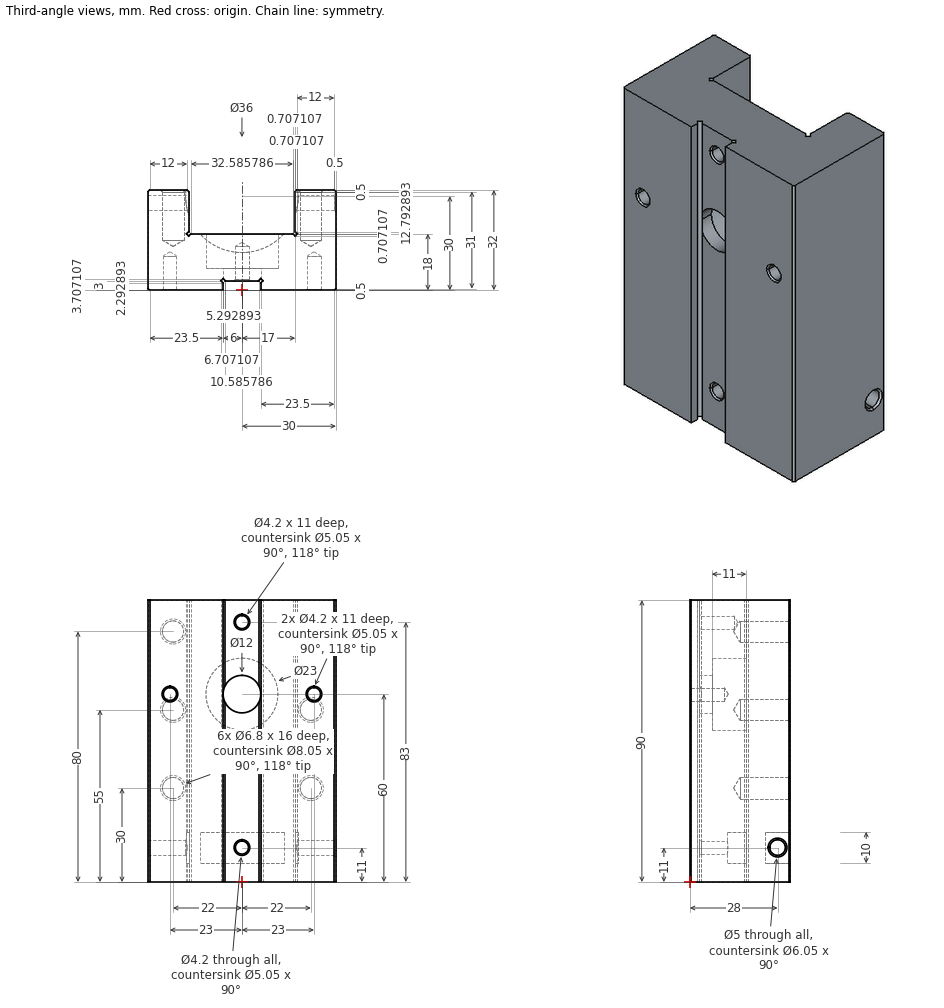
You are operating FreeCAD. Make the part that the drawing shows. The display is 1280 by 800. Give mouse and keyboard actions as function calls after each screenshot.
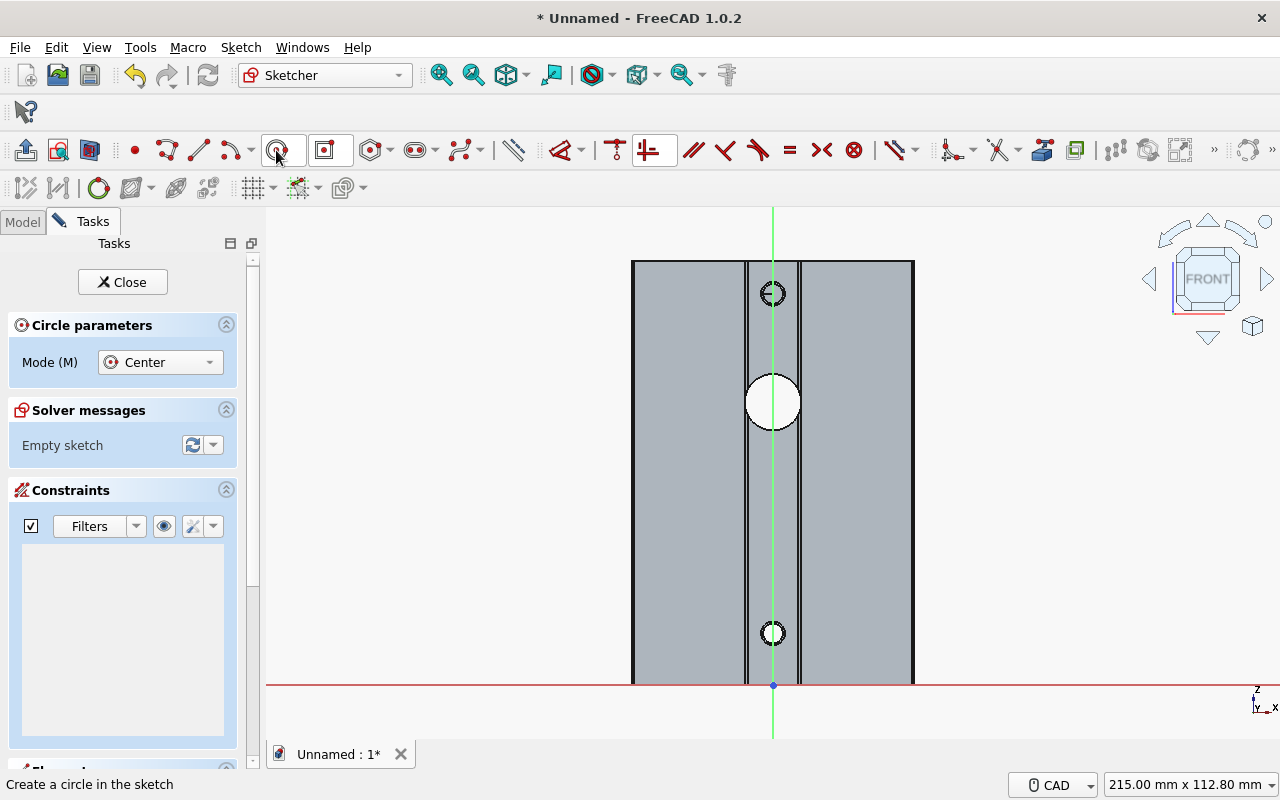
scroll(881, 402, up, 5)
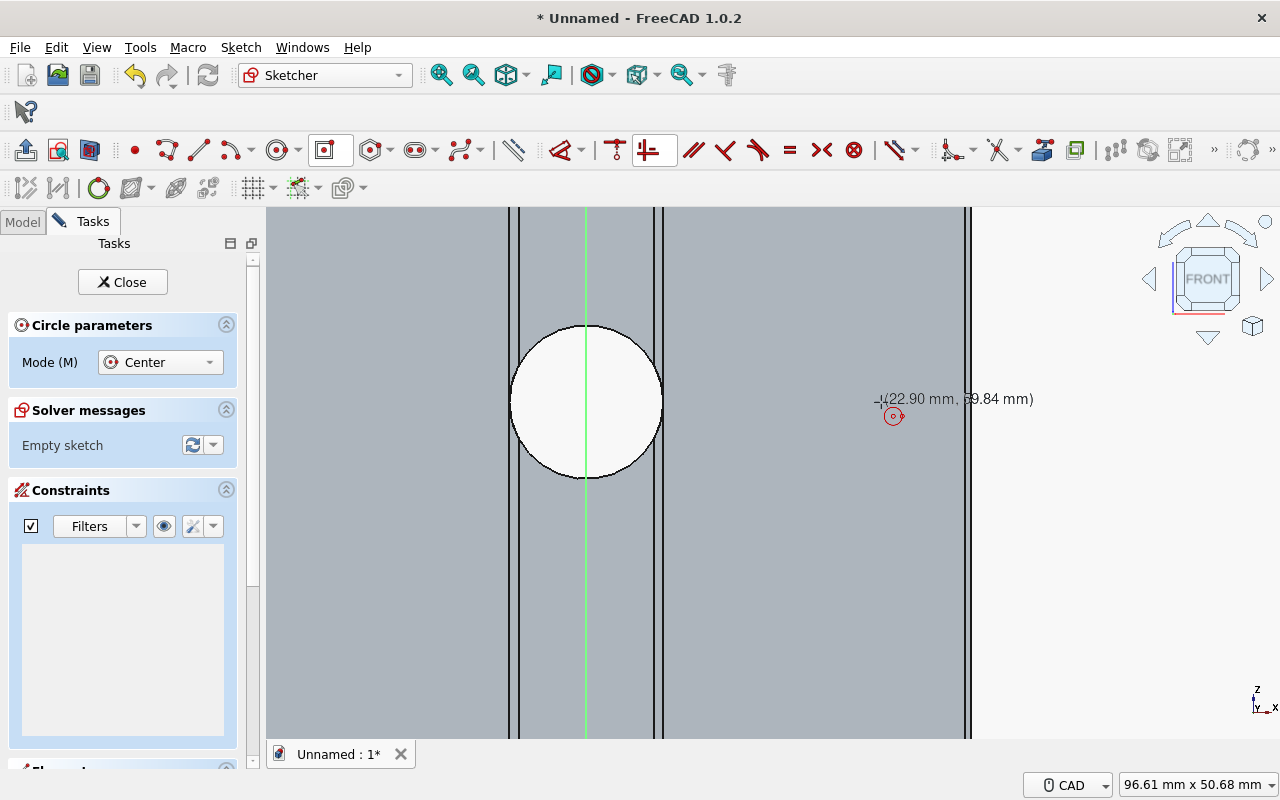
click(881, 402)
move(900, 383)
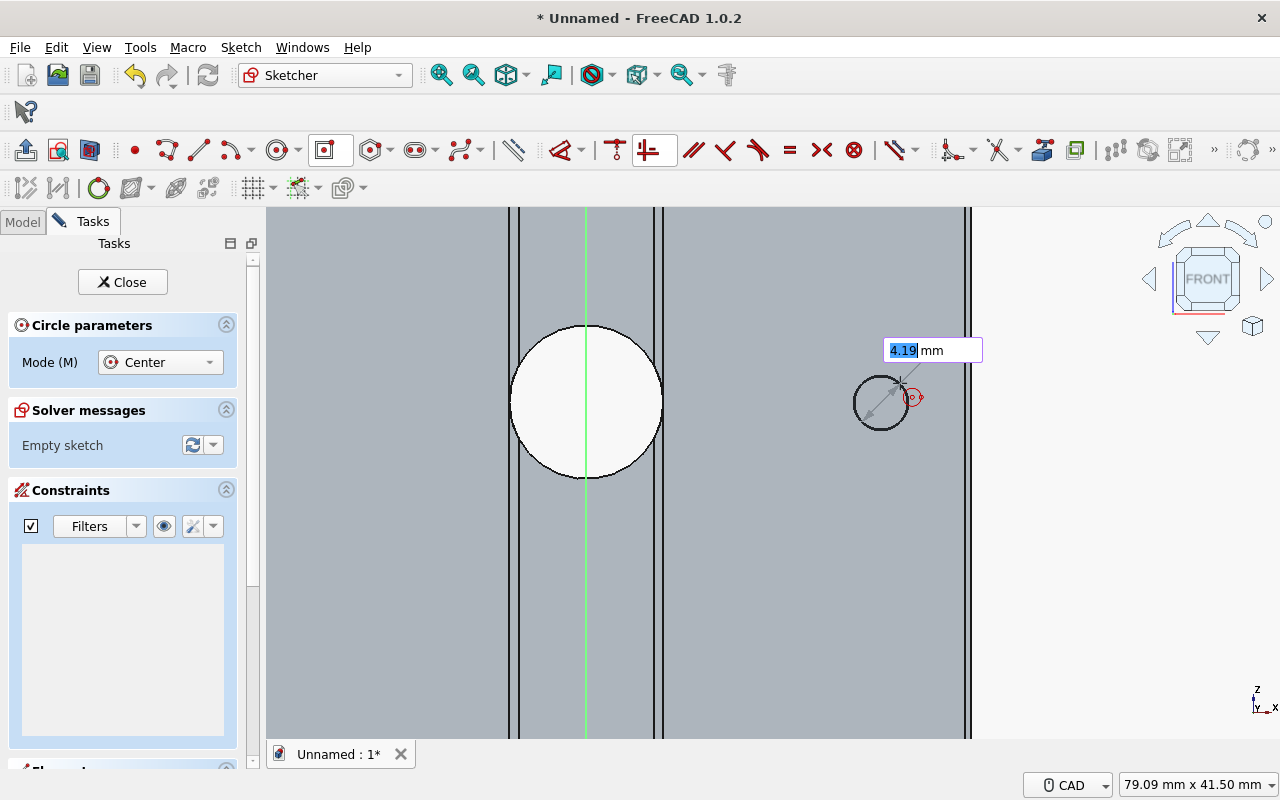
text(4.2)
key(Return)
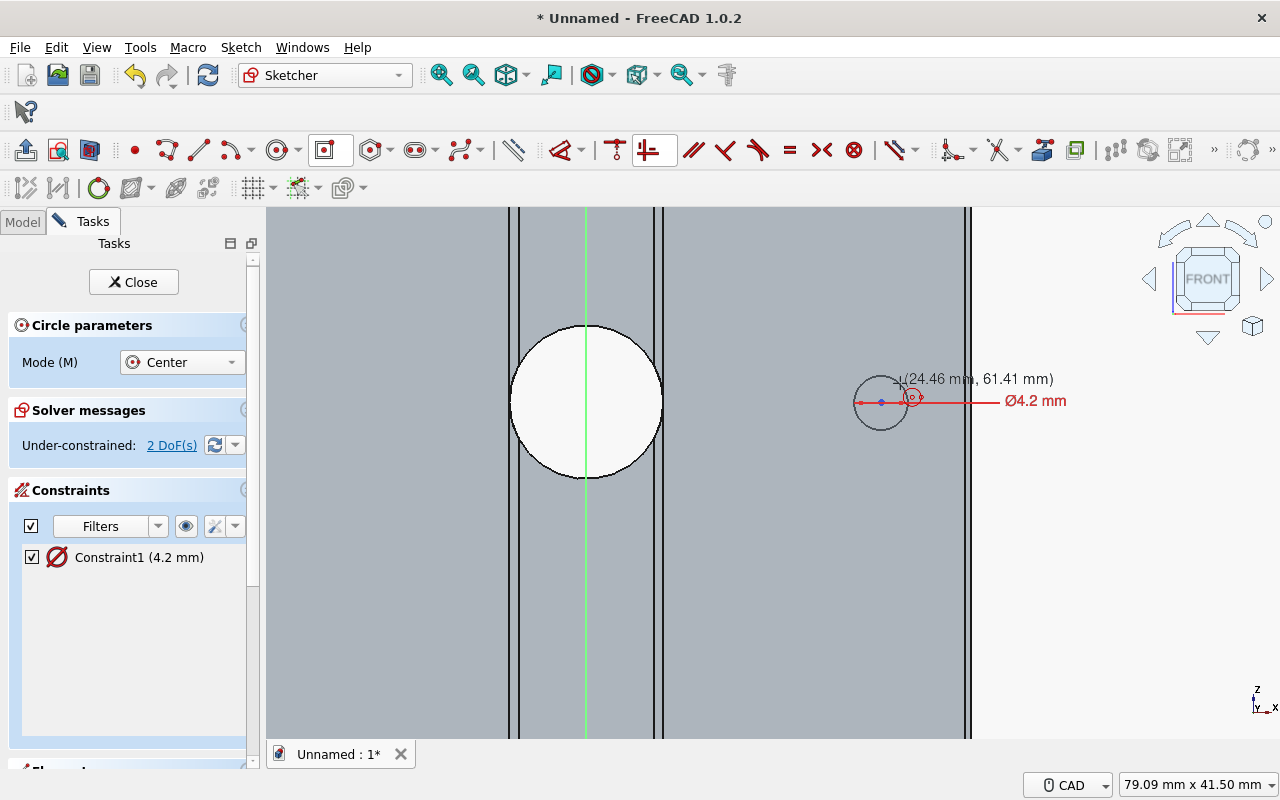
scroll(801, 235, down, 4)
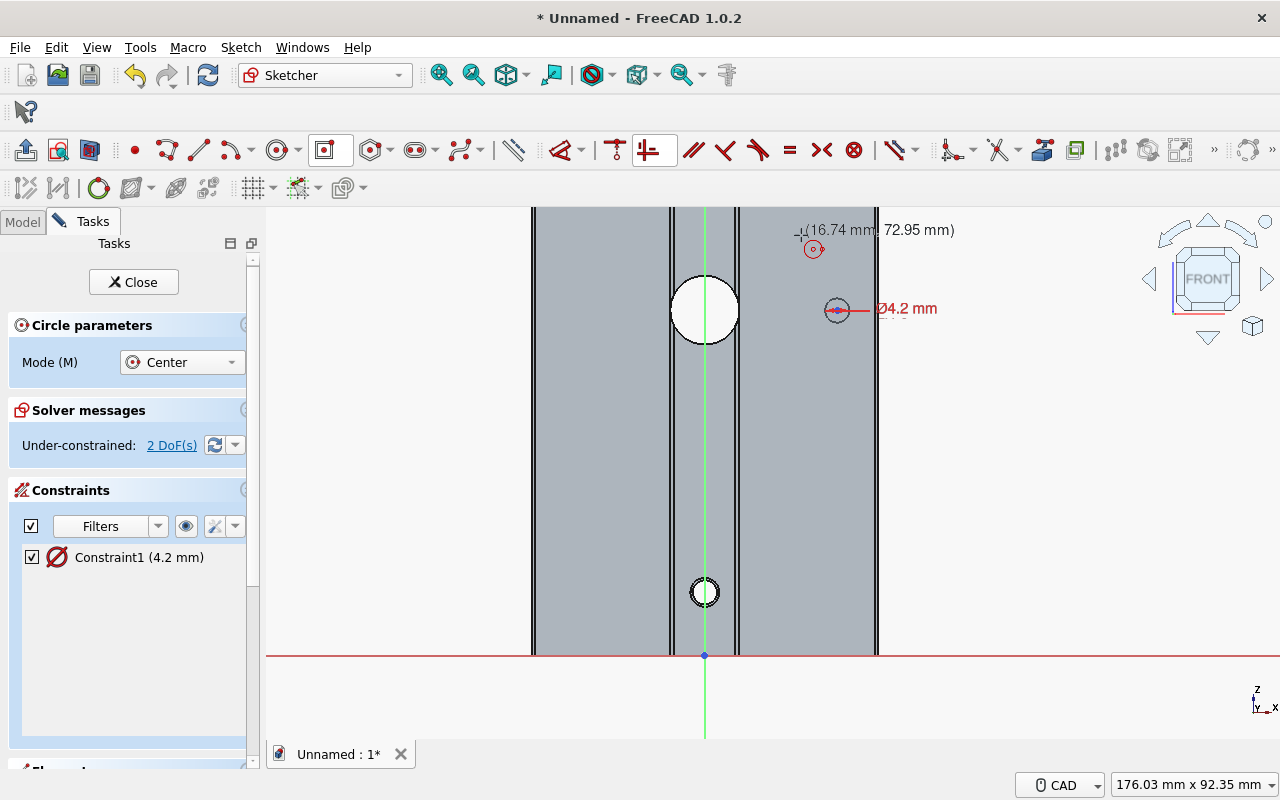
scroll(572, 310, up, 4)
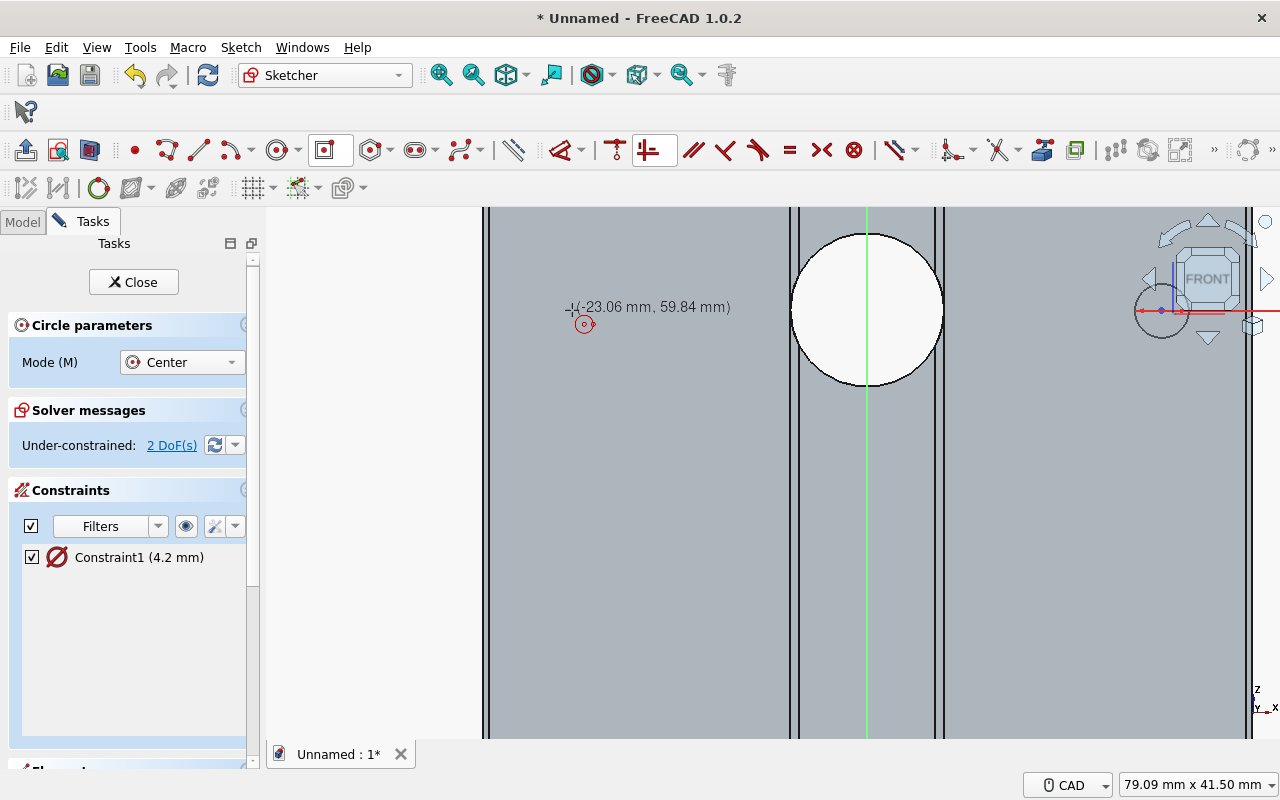
click(572, 310)
move(591, 291)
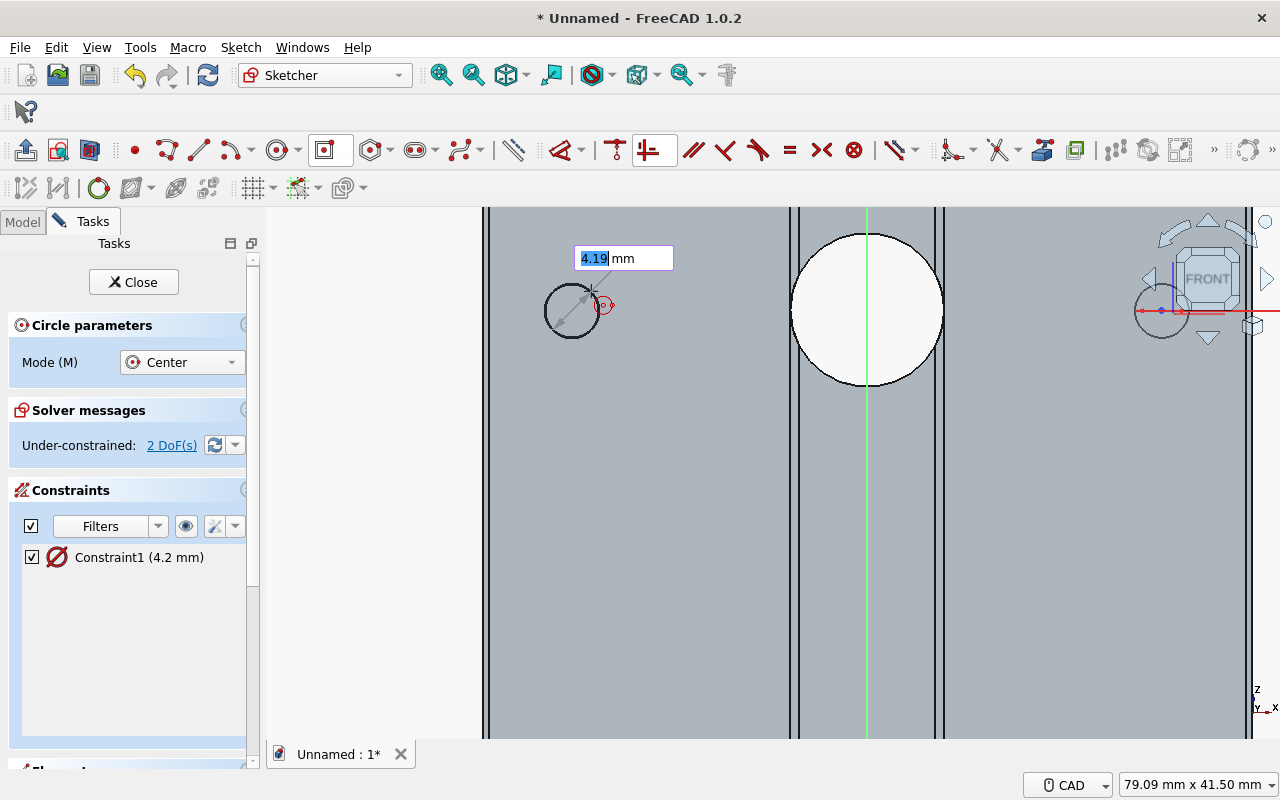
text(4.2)
key(Return)
key(Escape)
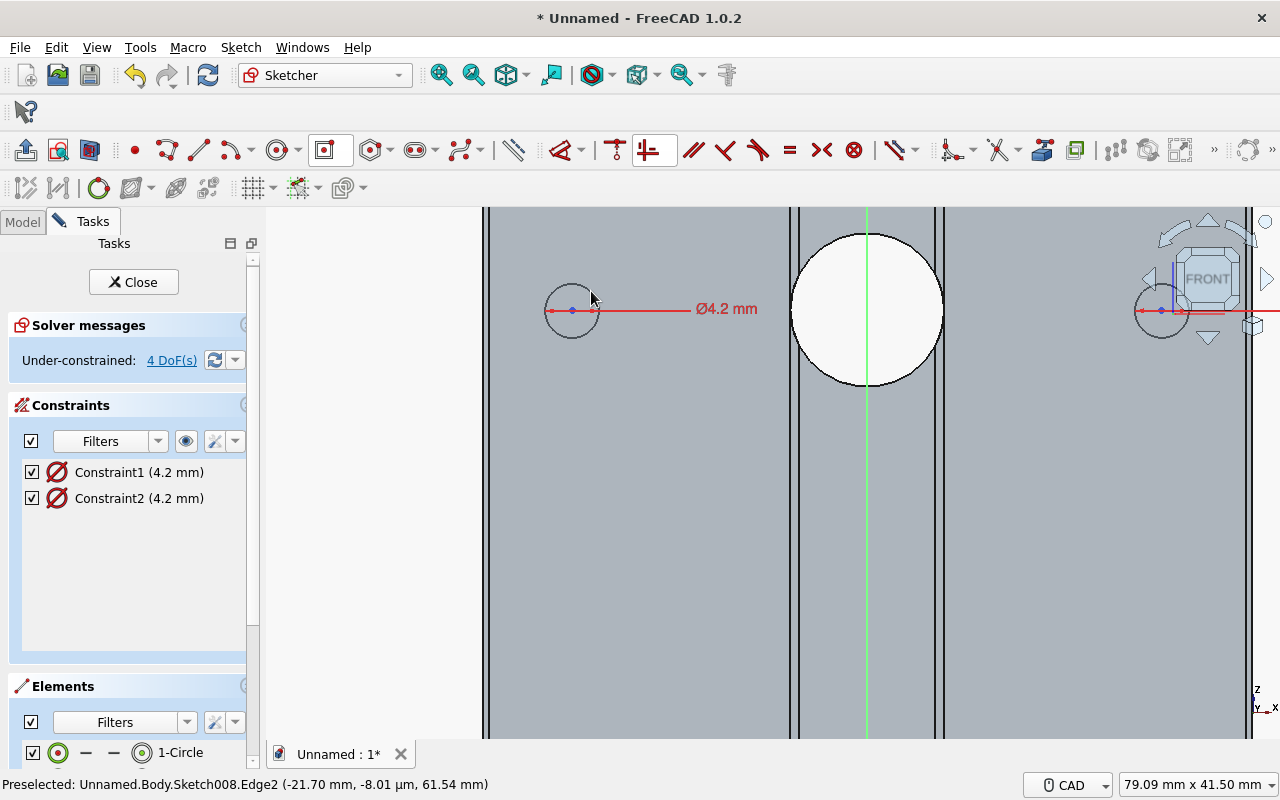
scroll(572, 303, down, 4)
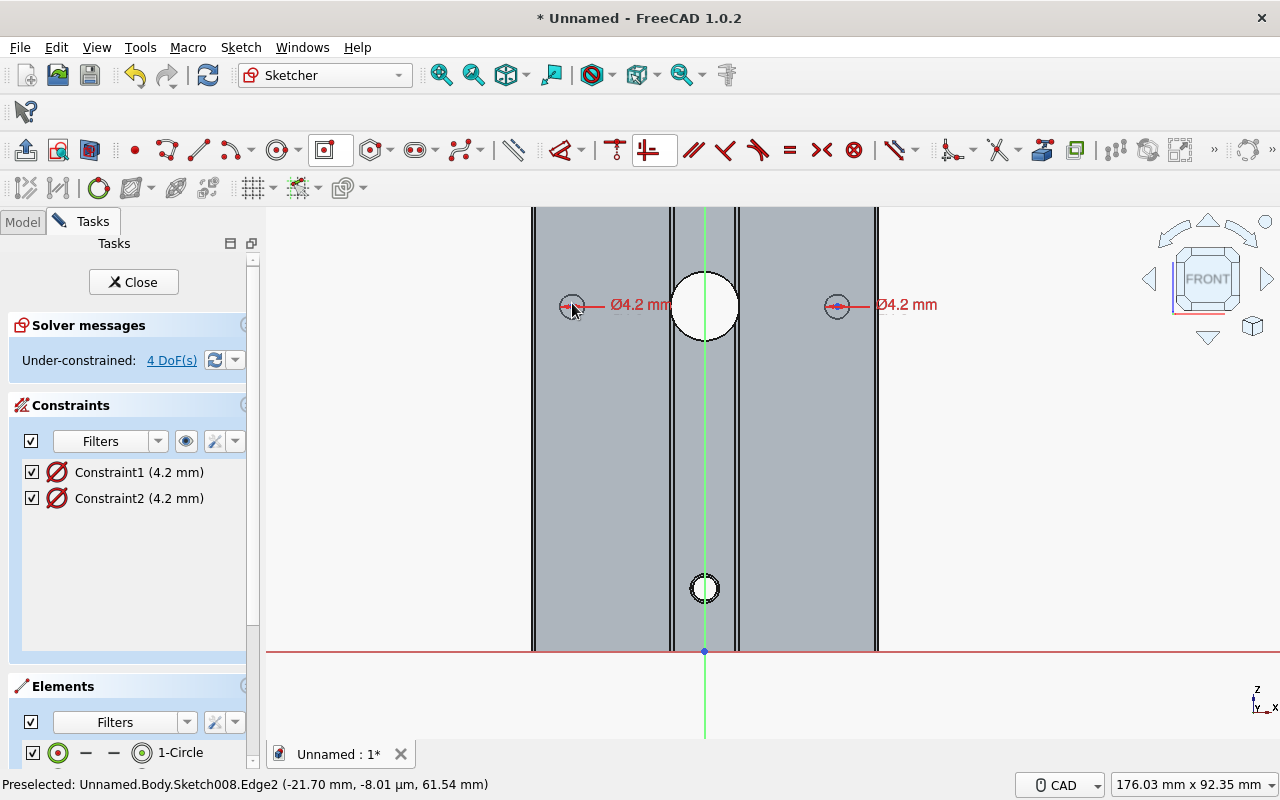
click(837, 307)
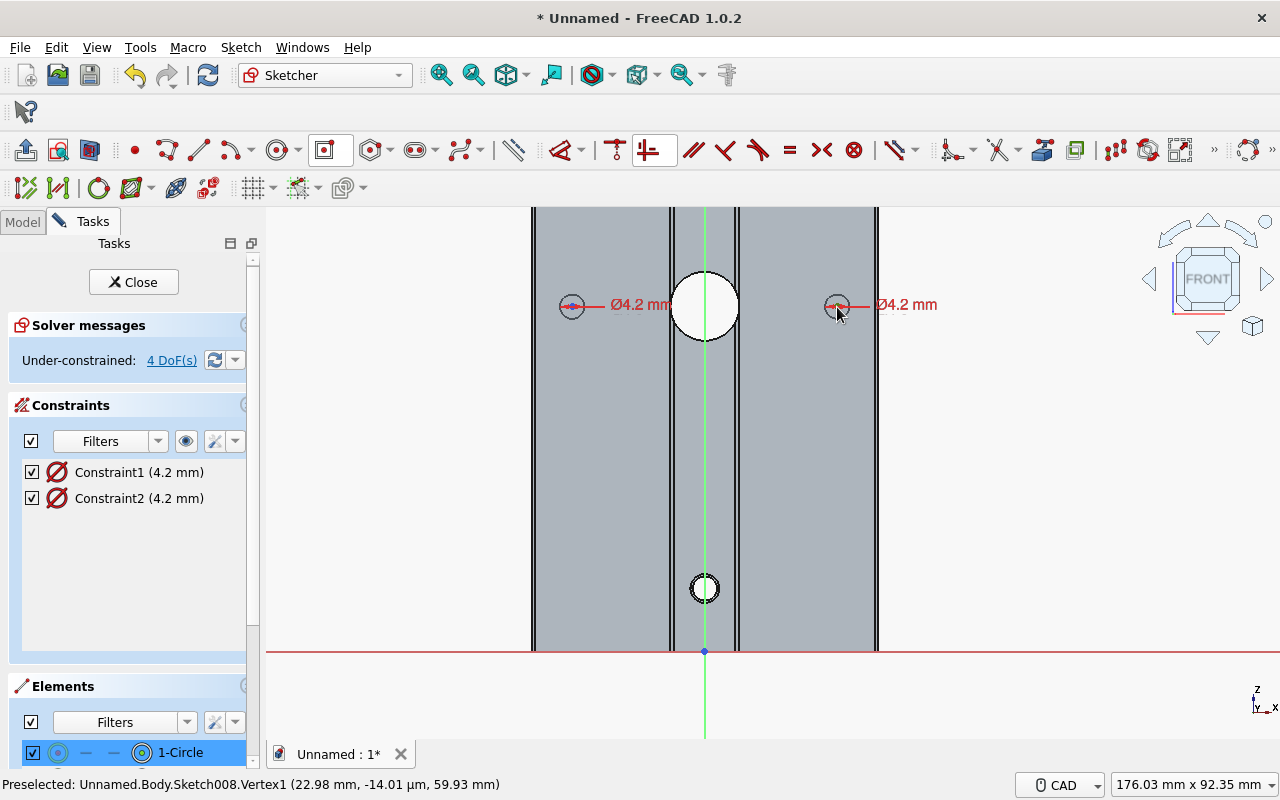
click(572, 307)